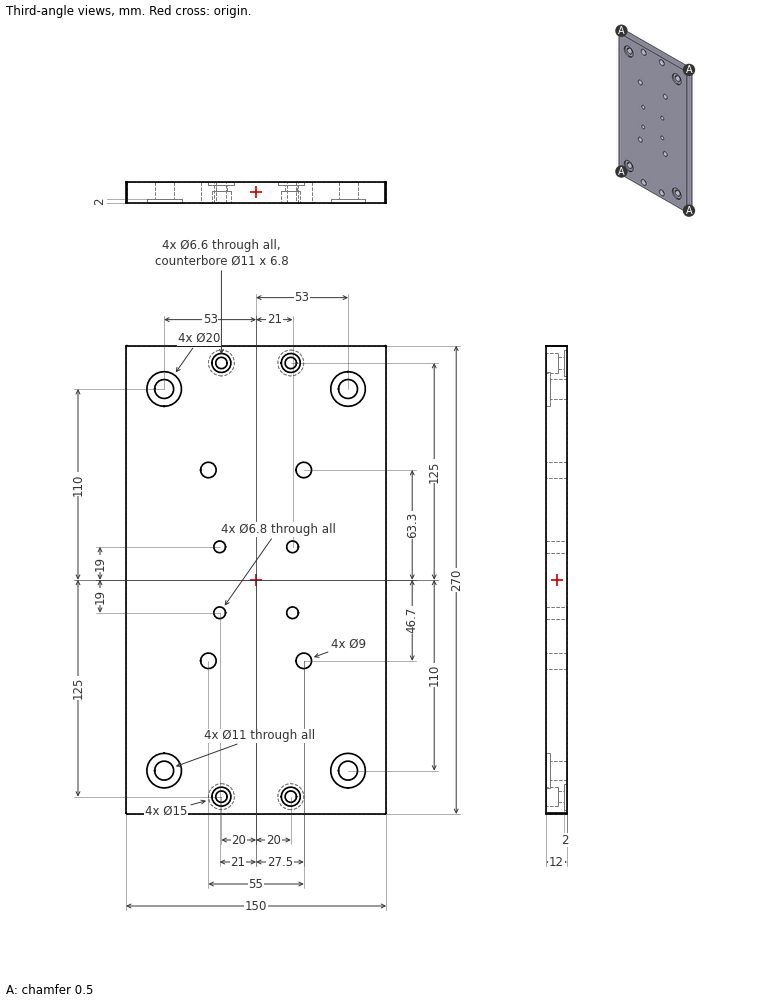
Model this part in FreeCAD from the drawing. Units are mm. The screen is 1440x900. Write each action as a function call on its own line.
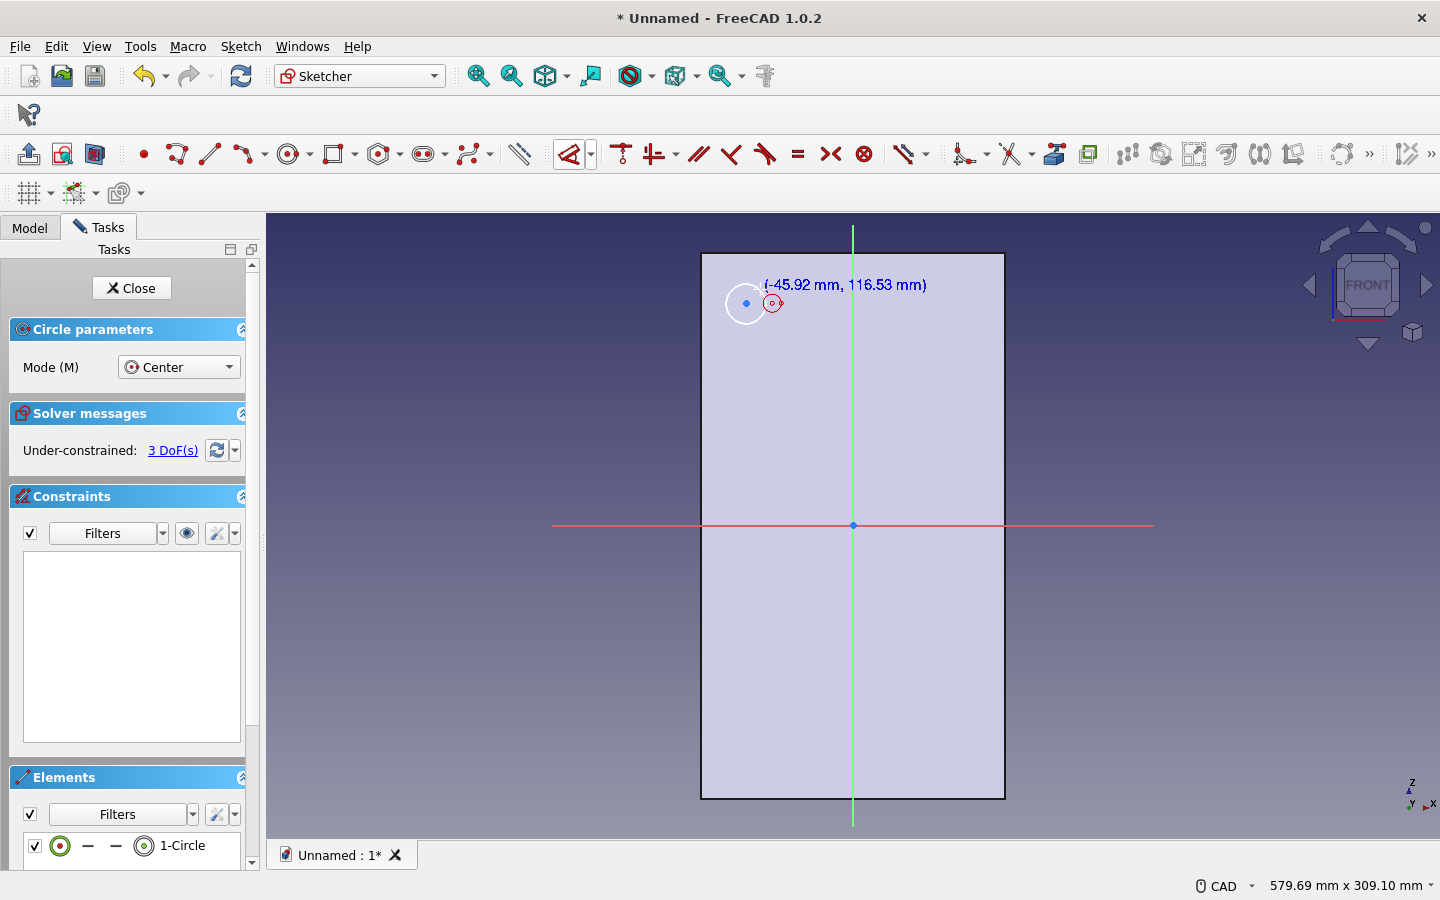
click(960, 303)
click(975, 289)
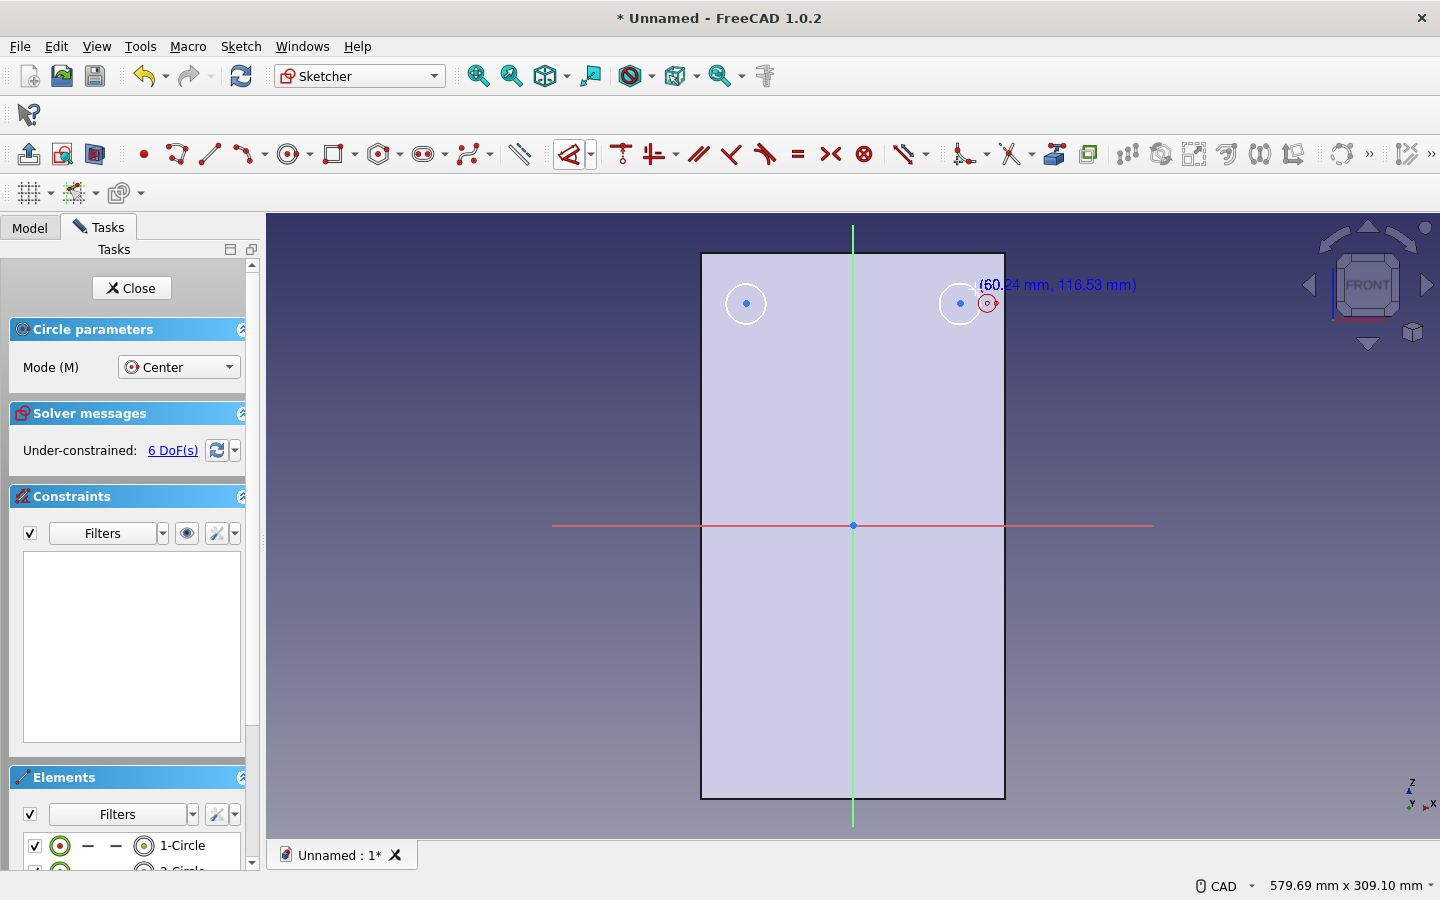
click(960, 749)
click(975, 734)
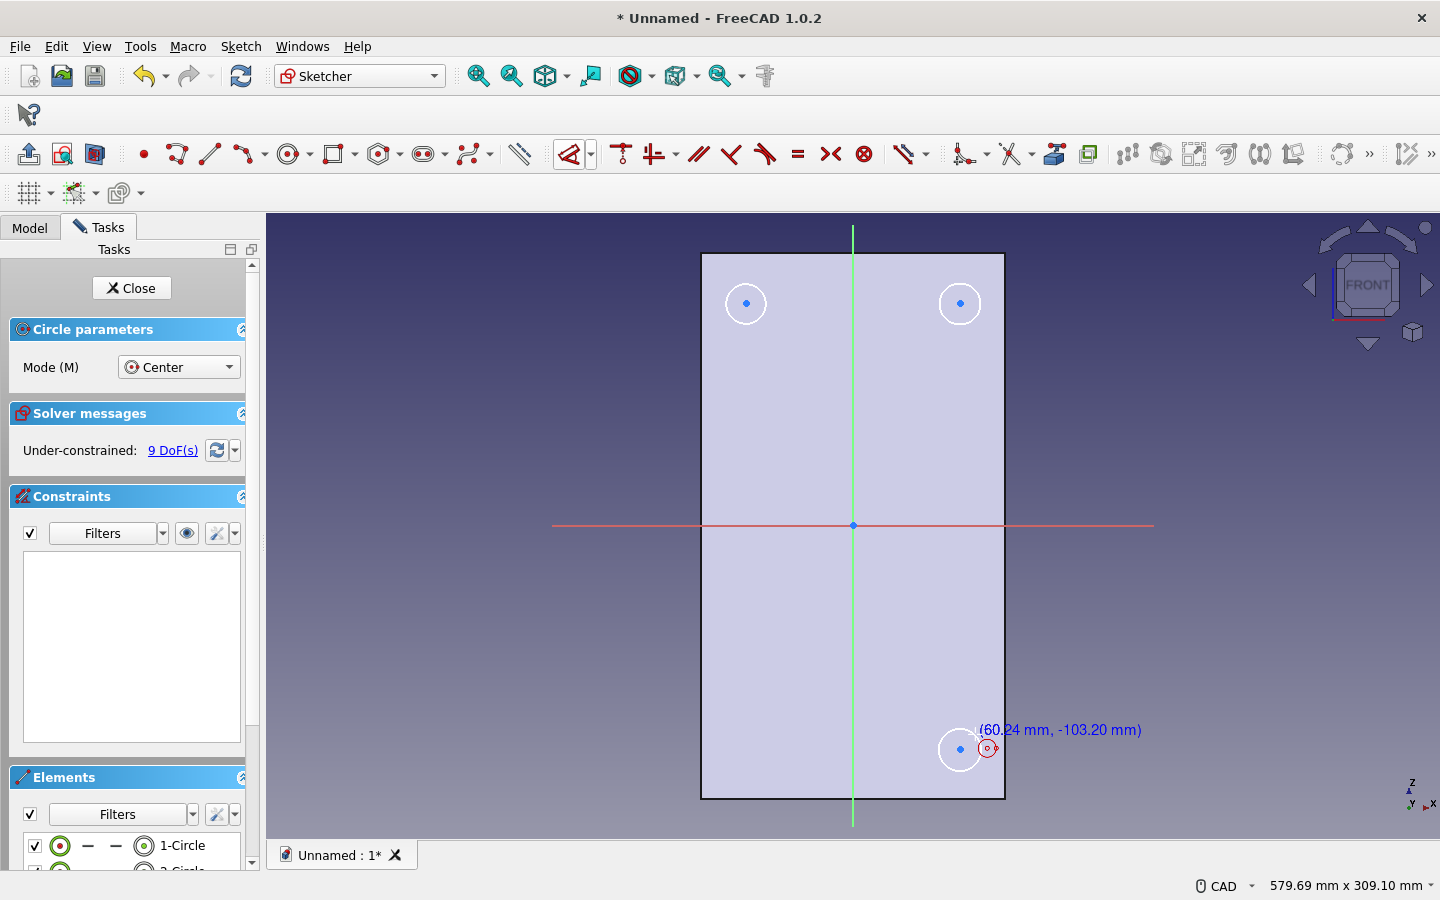
click(746, 749)
click(760, 734)
key(Escape)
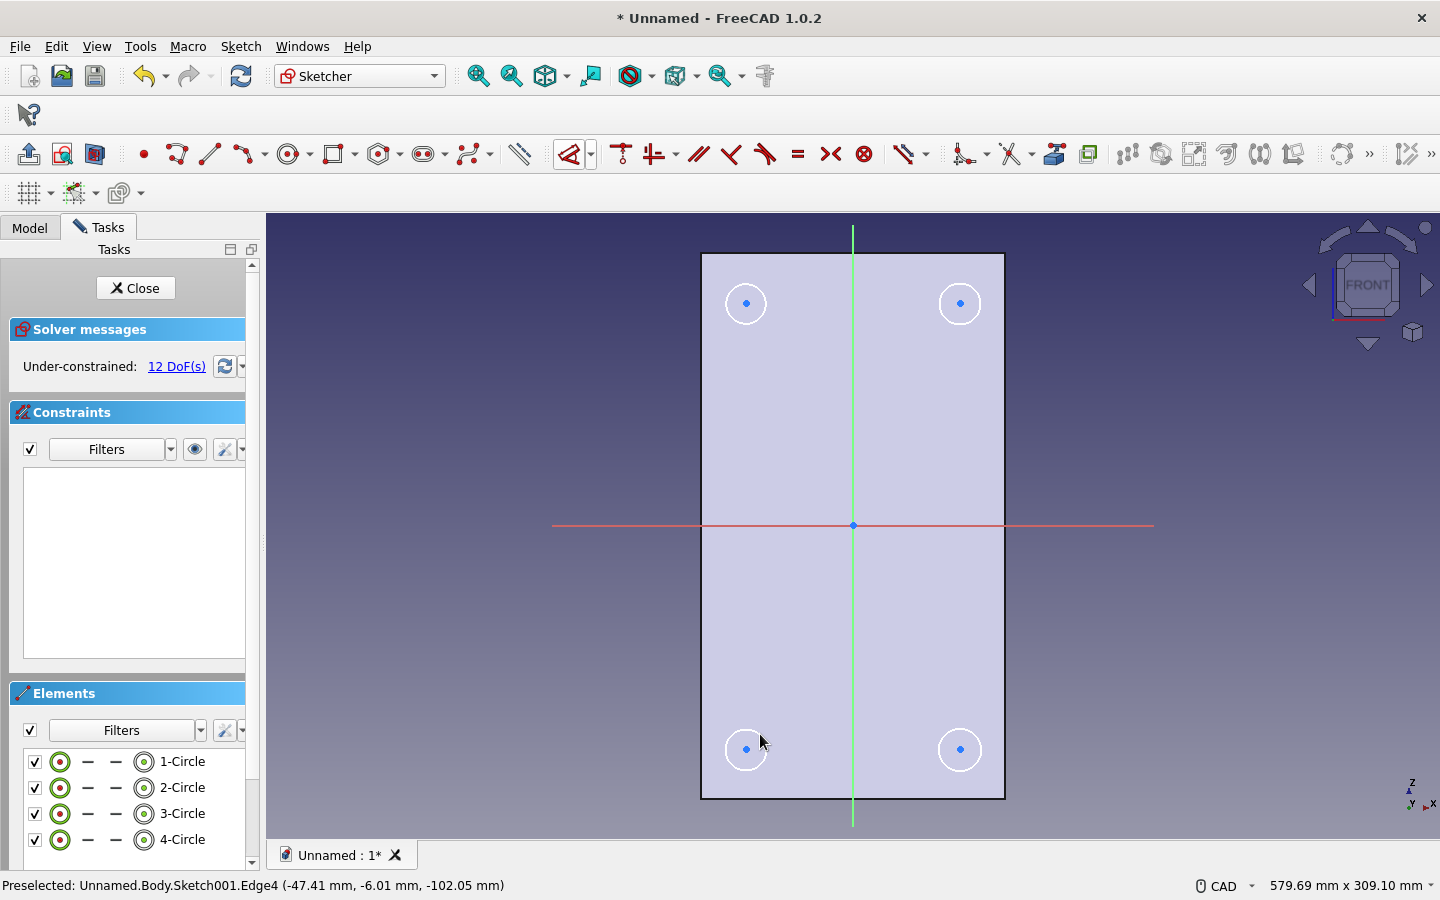
click(760, 290)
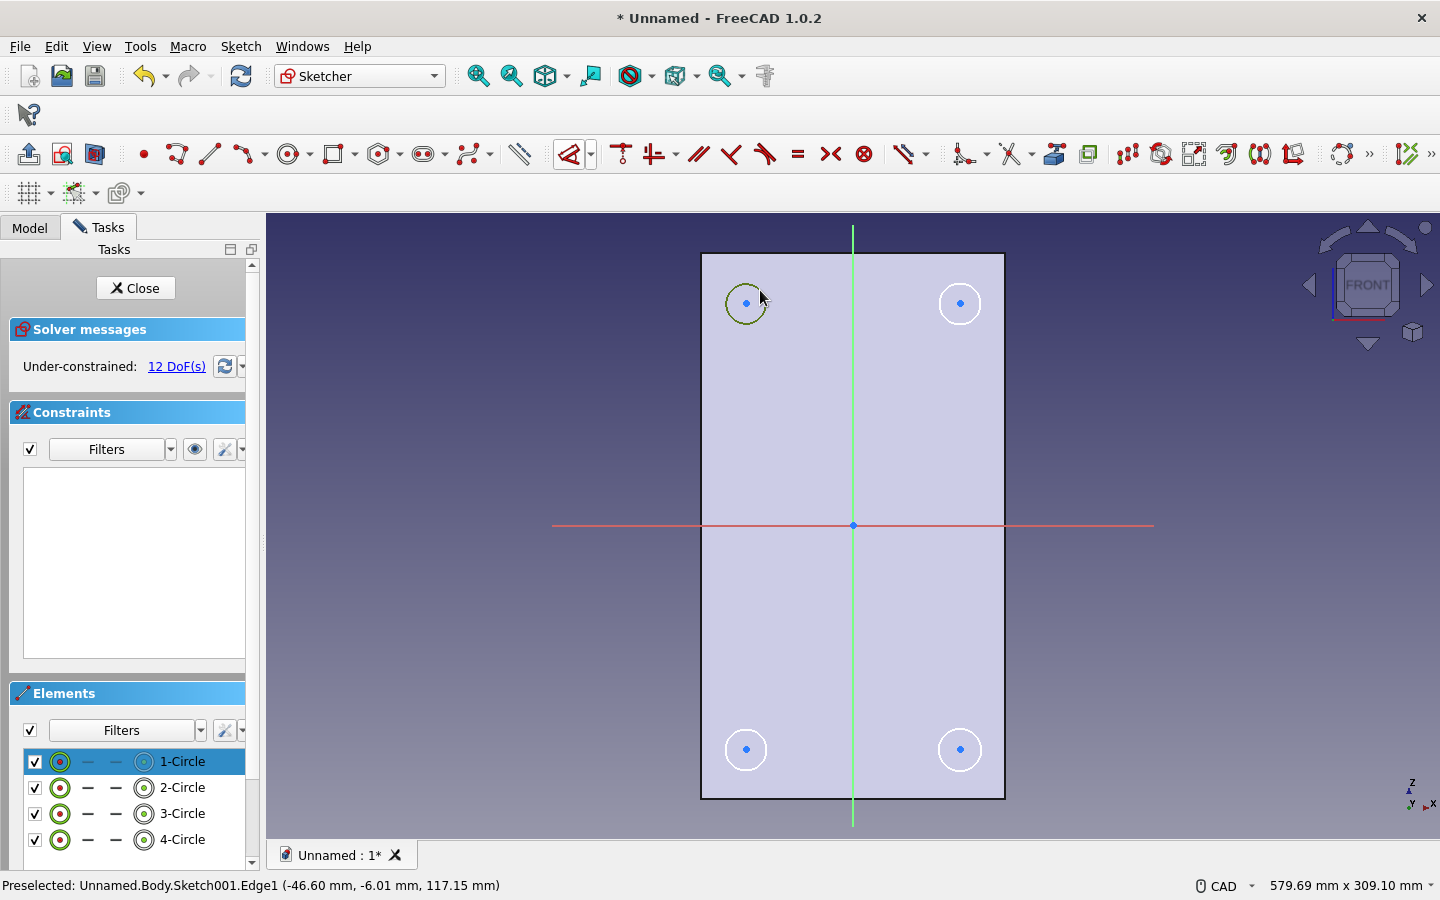
click(974, 289)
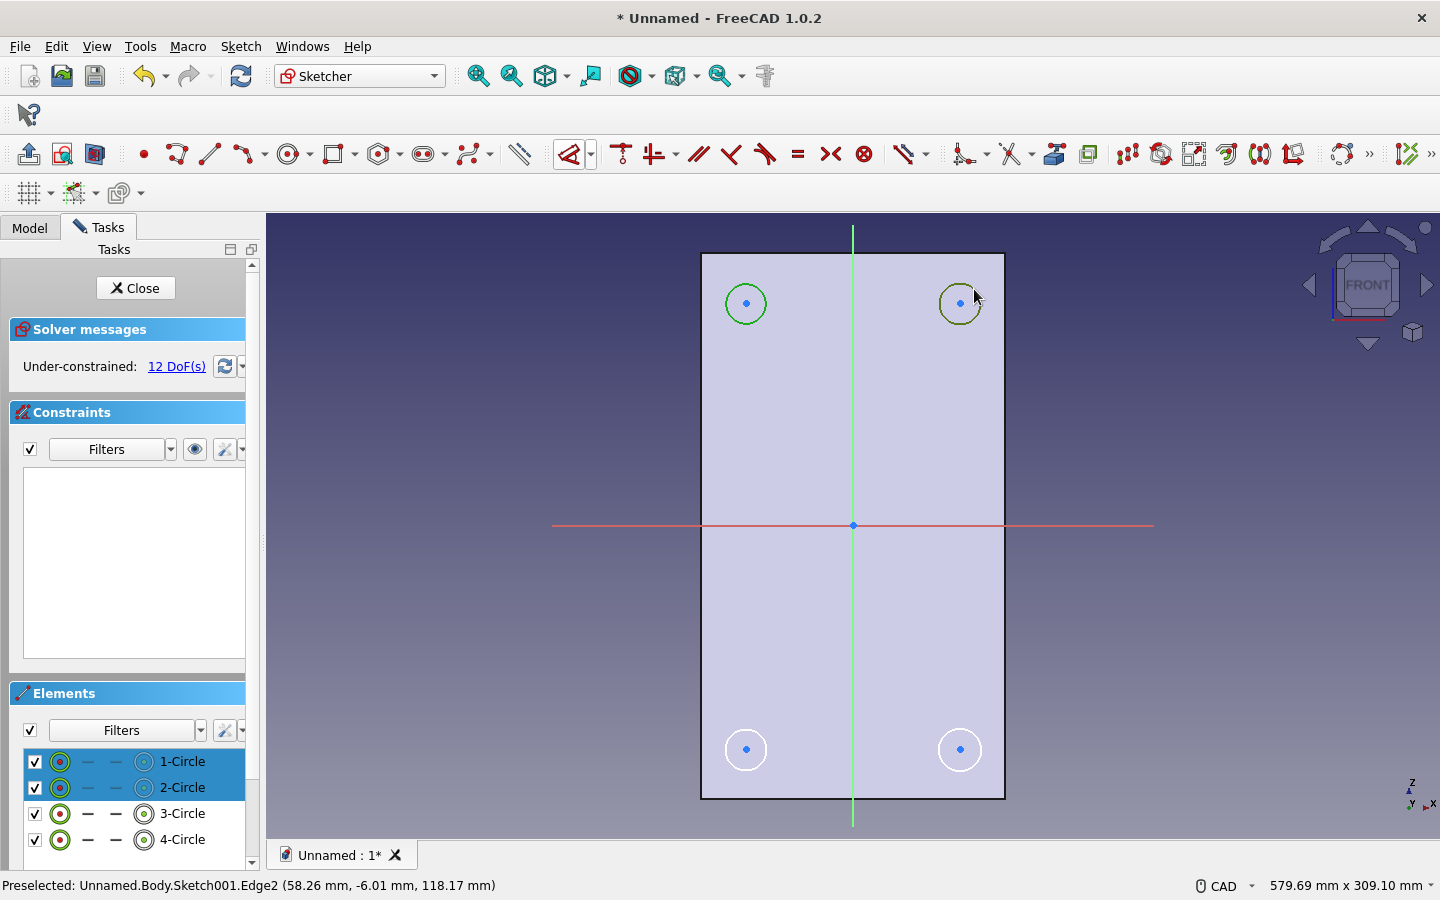
click(975, 735)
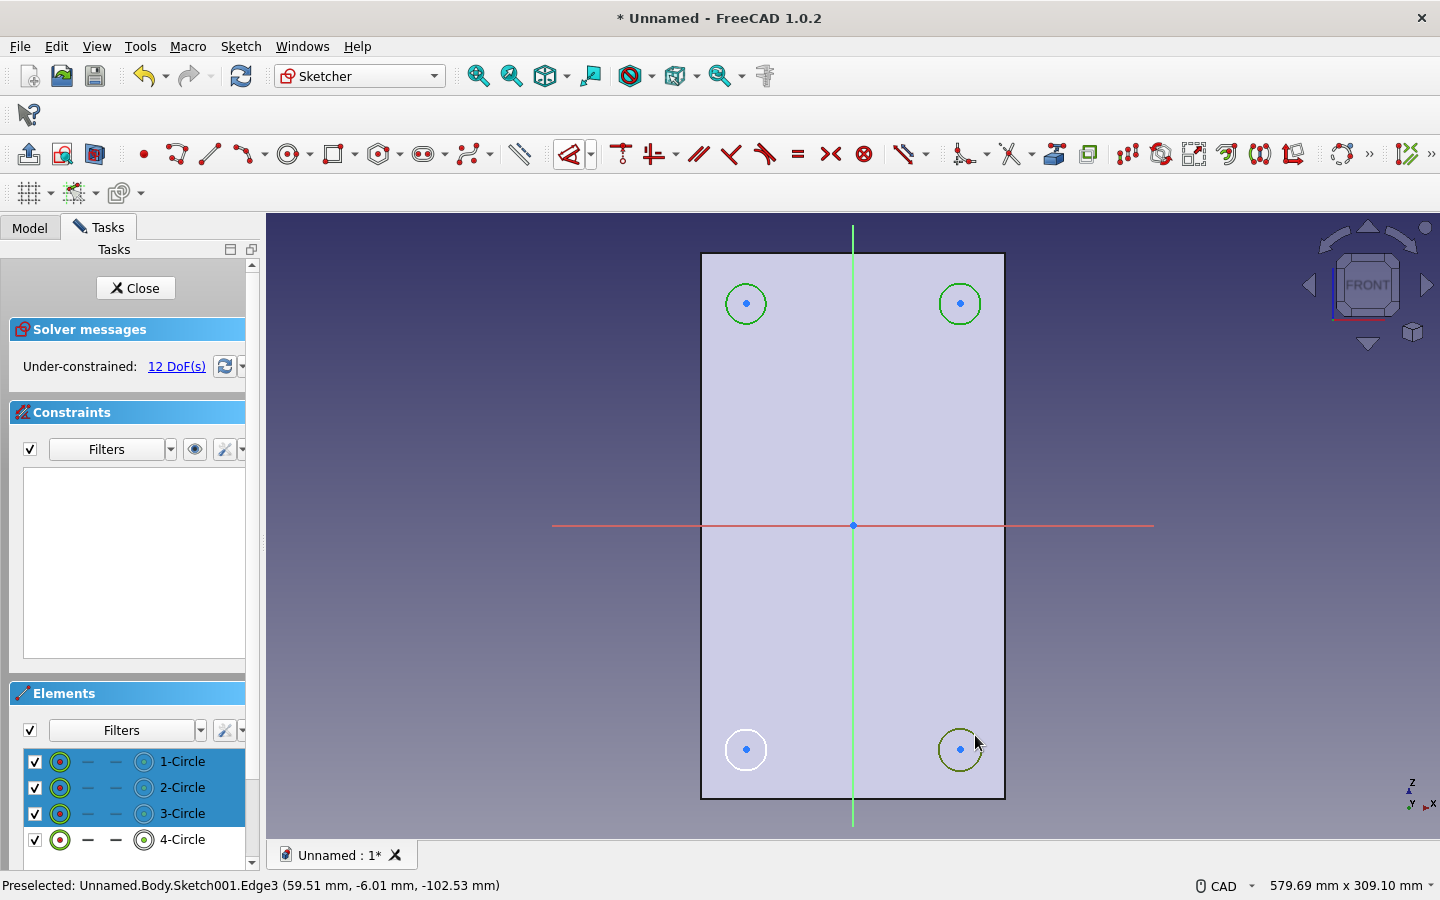
click(760, 735)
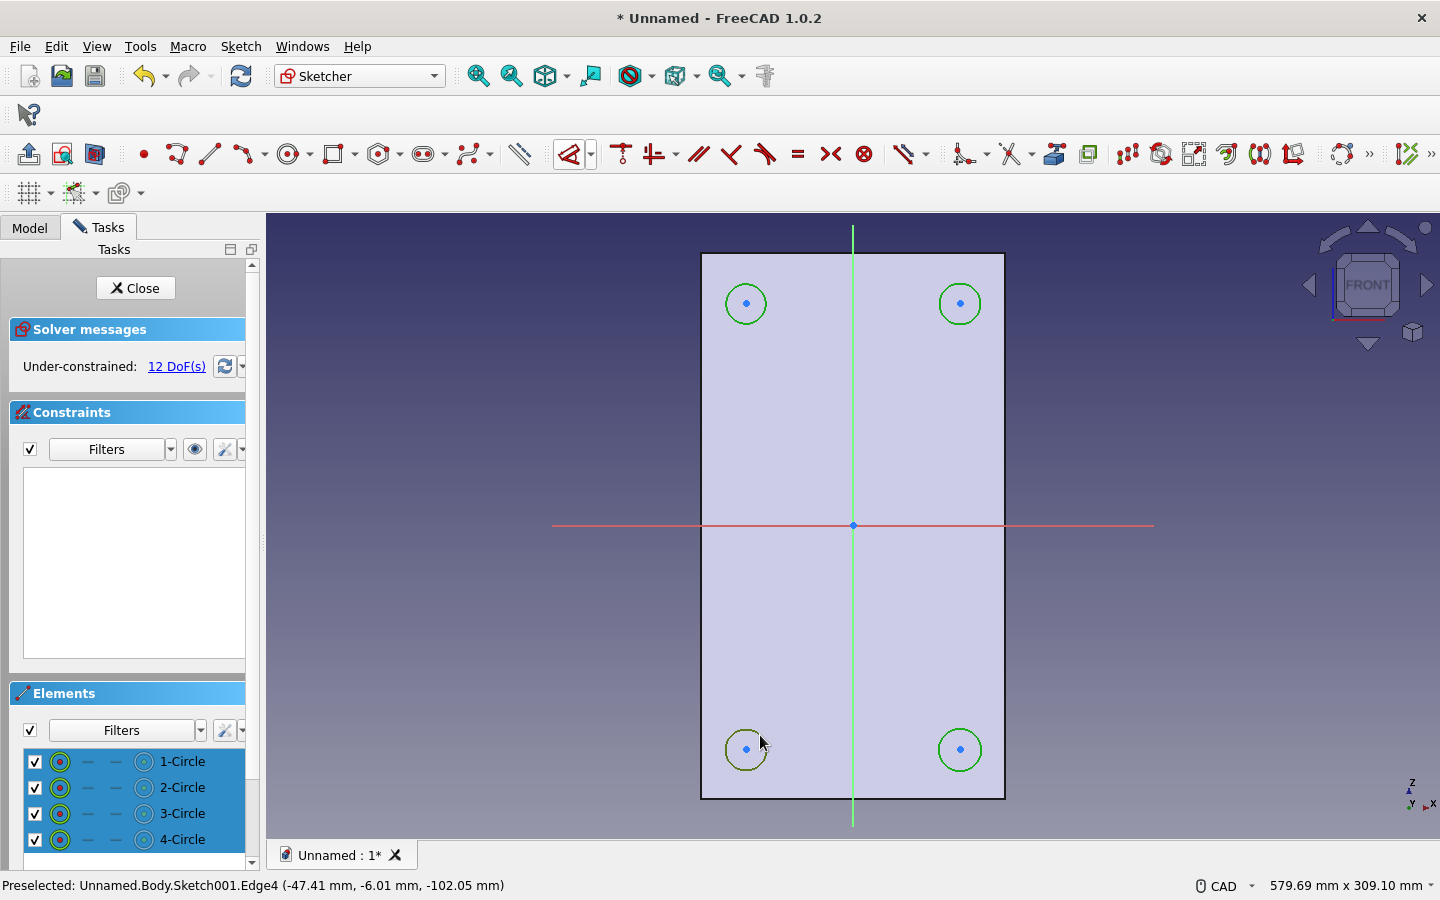
key(e)